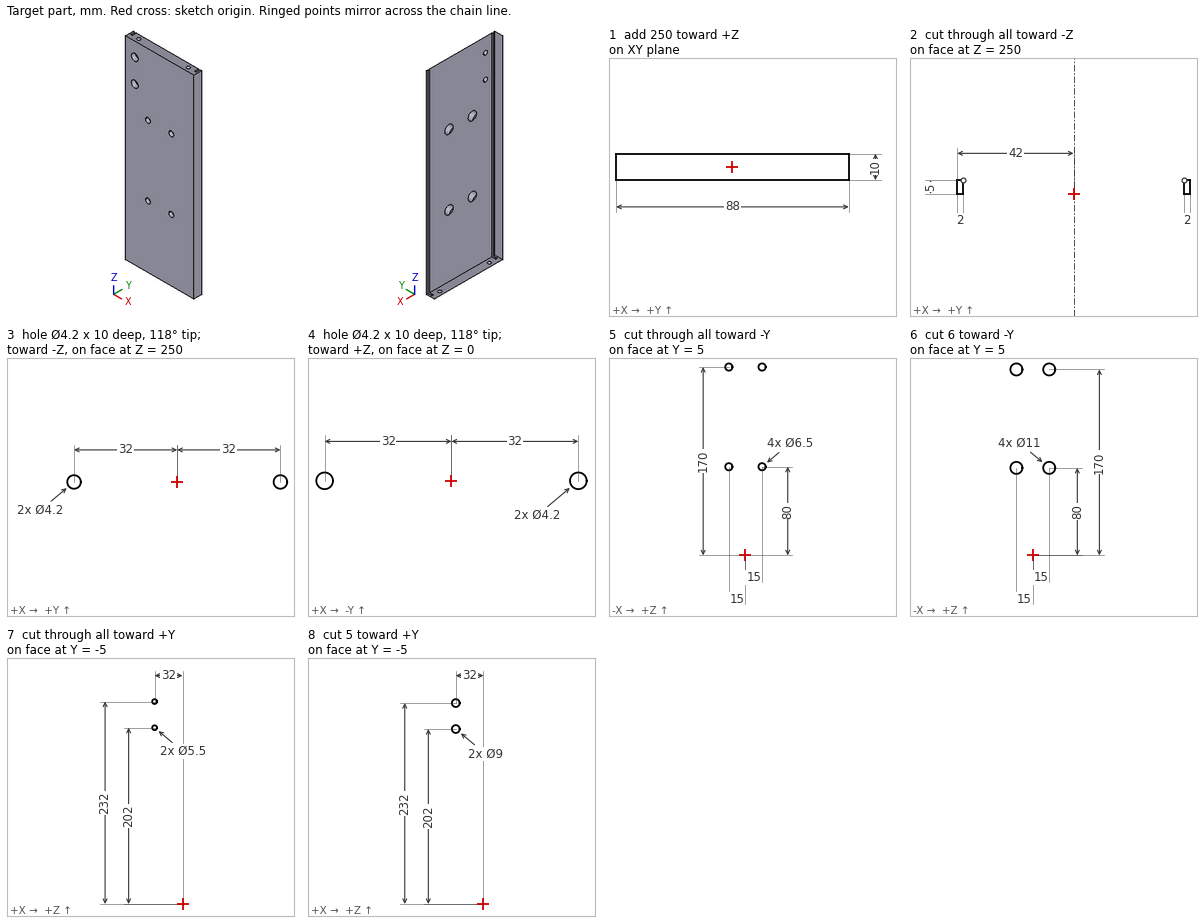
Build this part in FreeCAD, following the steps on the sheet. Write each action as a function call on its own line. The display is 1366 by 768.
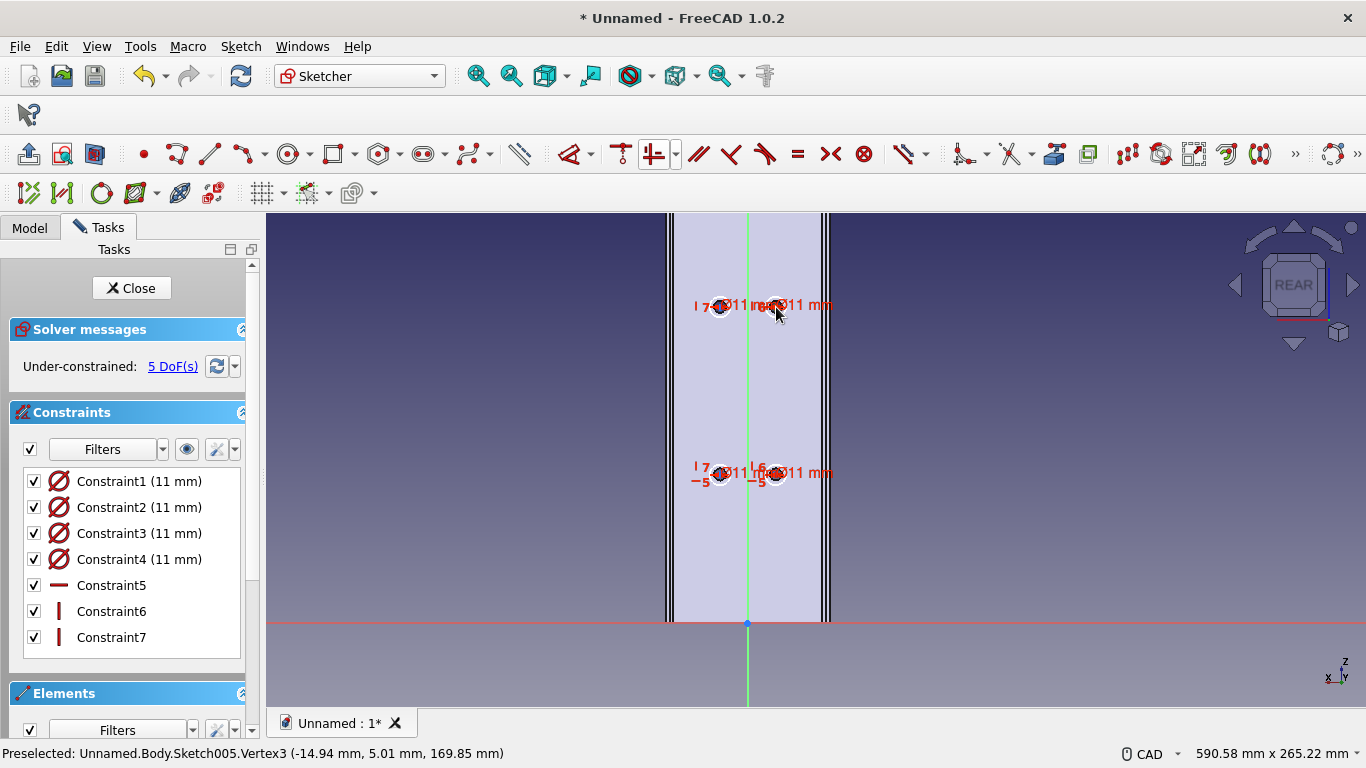
click(720, 307)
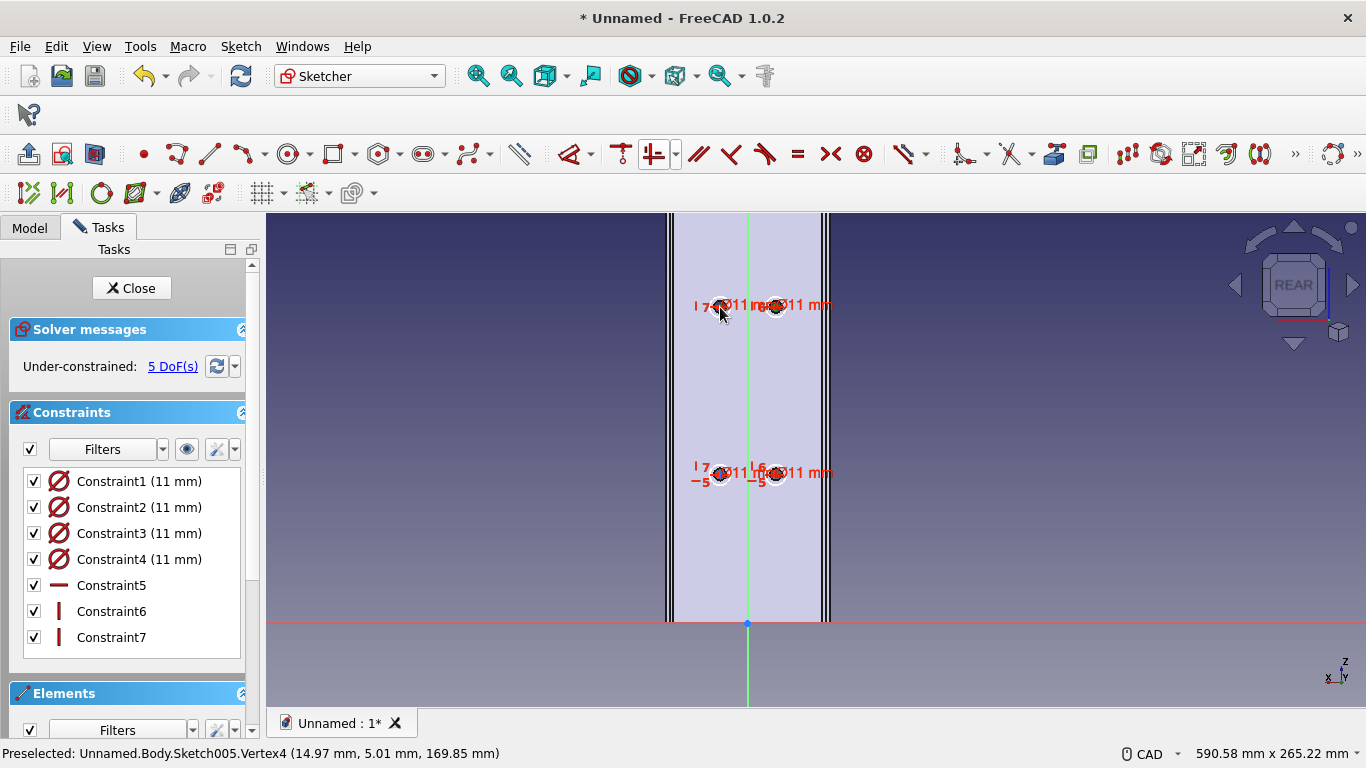
key(h)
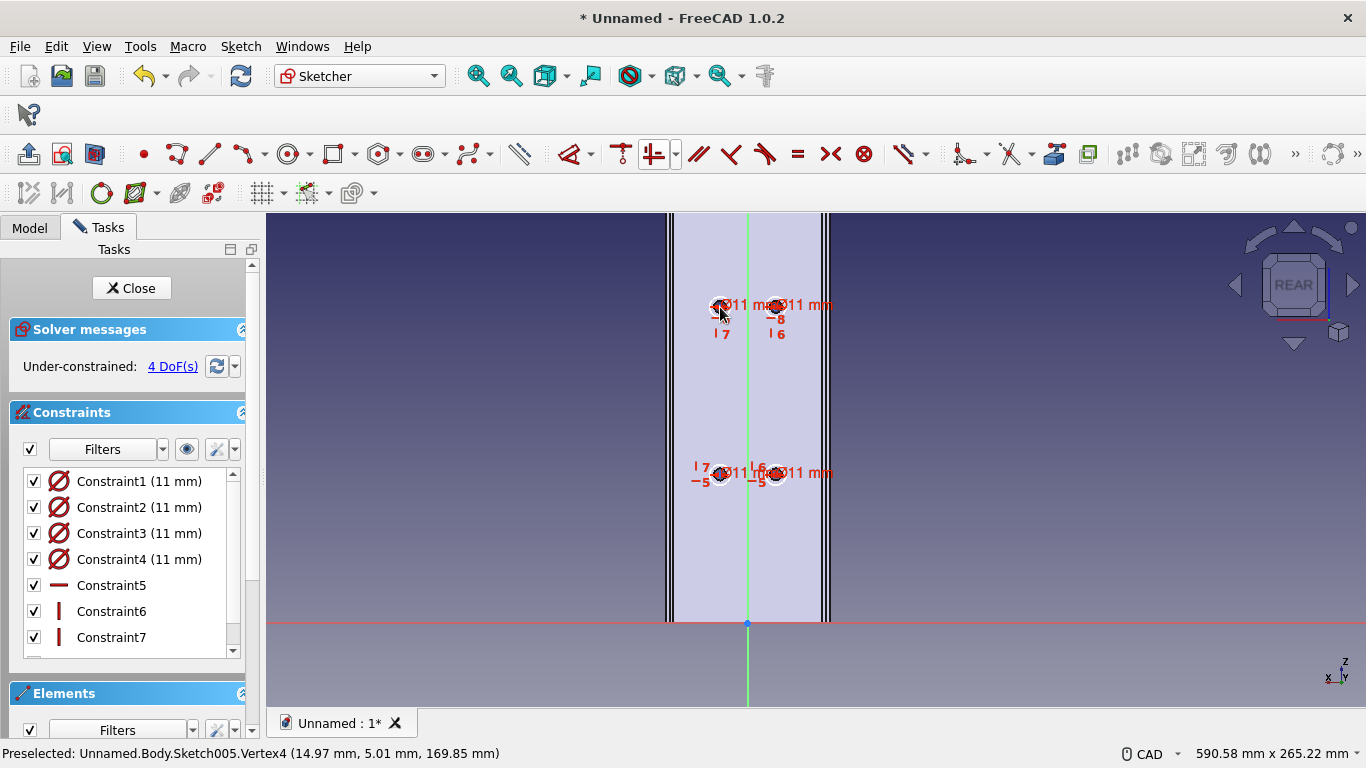
click(568, 154)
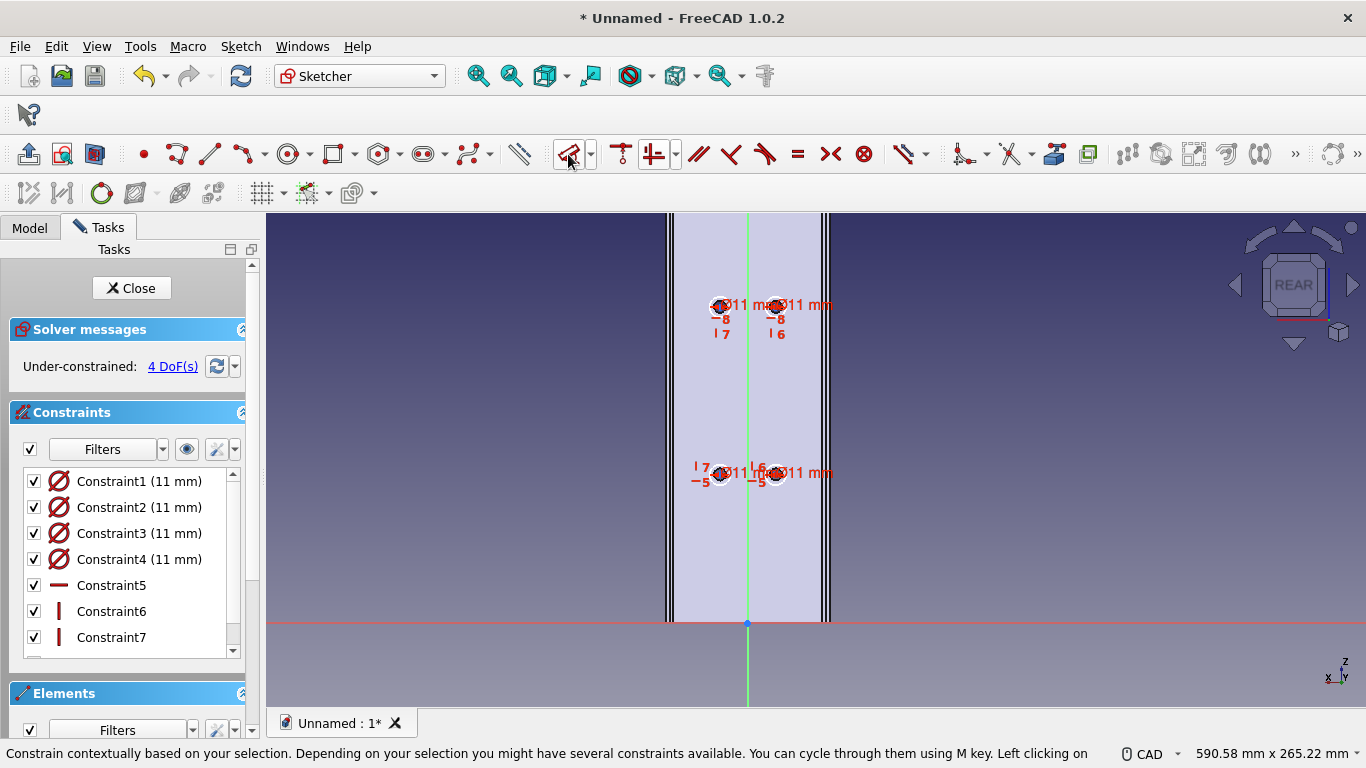
scroll(776, 475, up, 2)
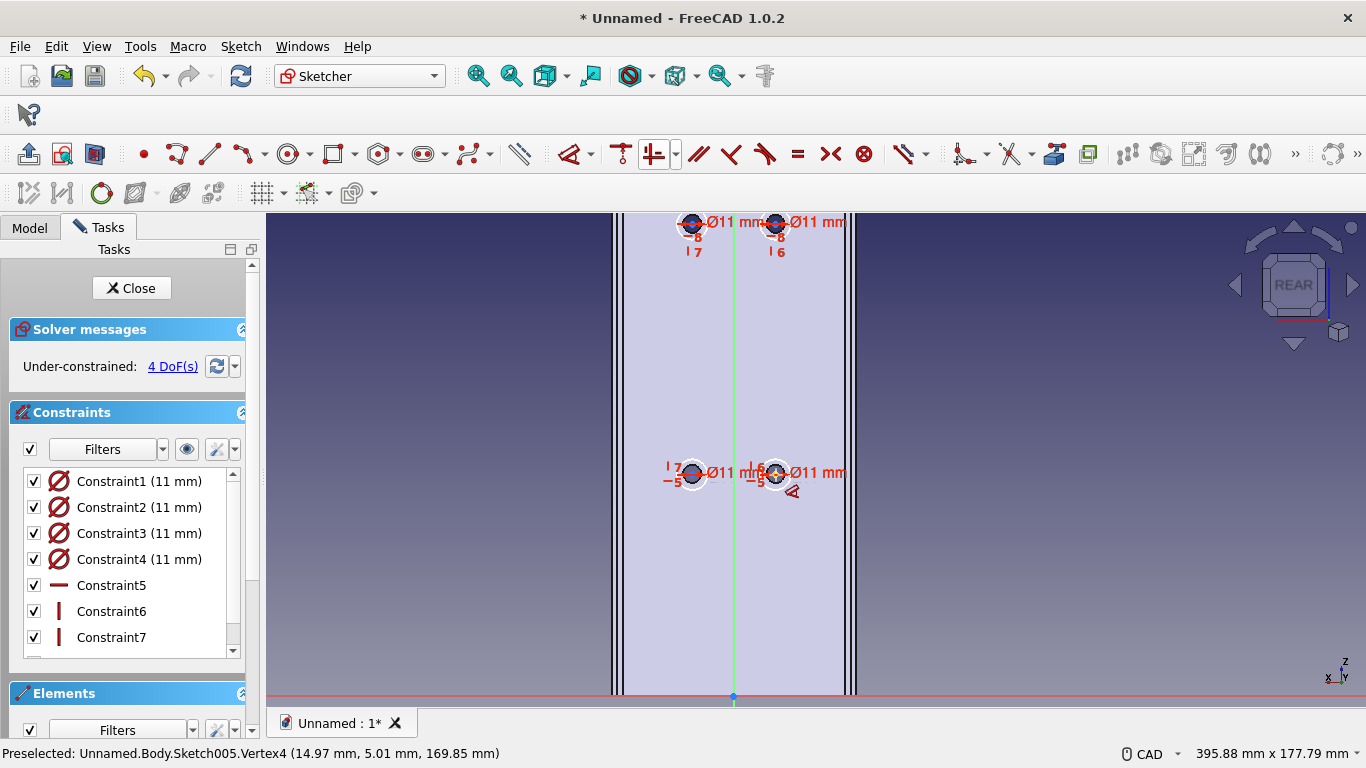
click(775, 475)
click(755, 441)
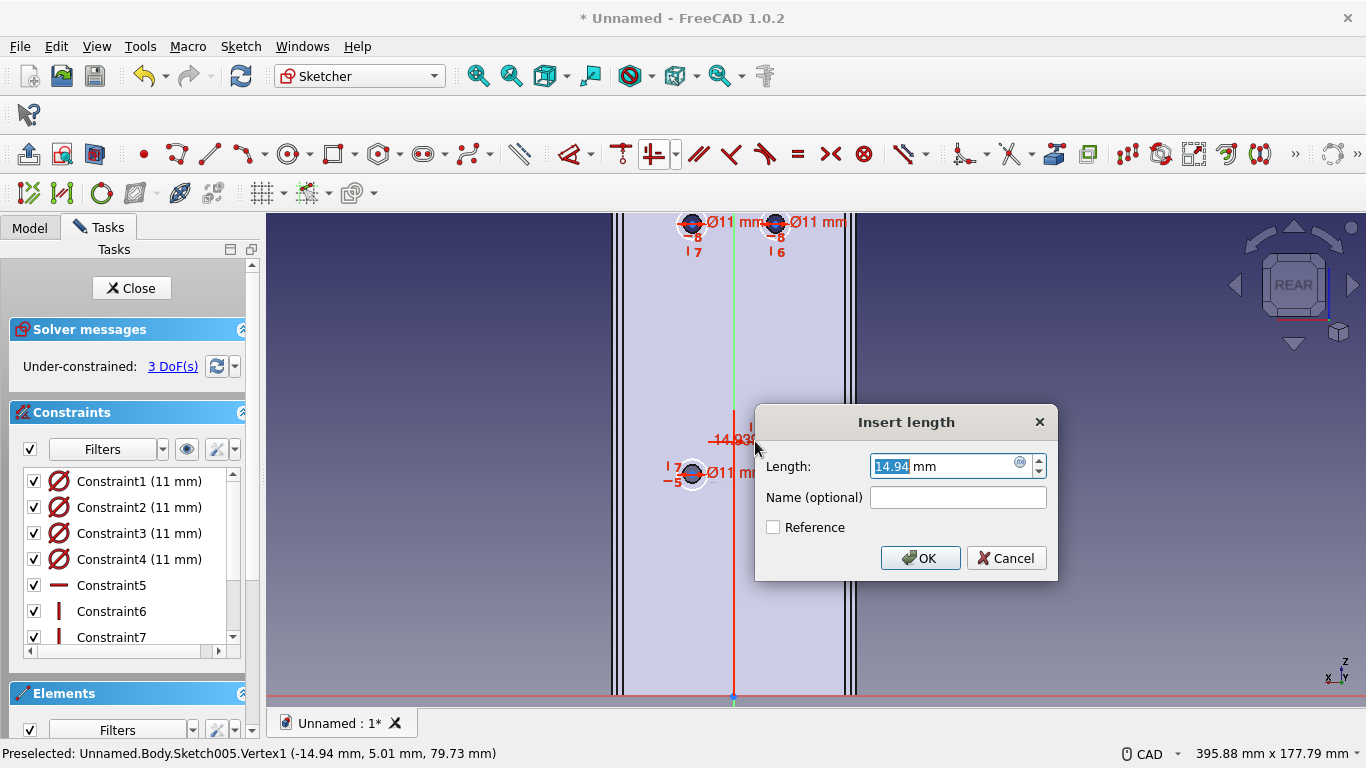
text(15)
key(Return)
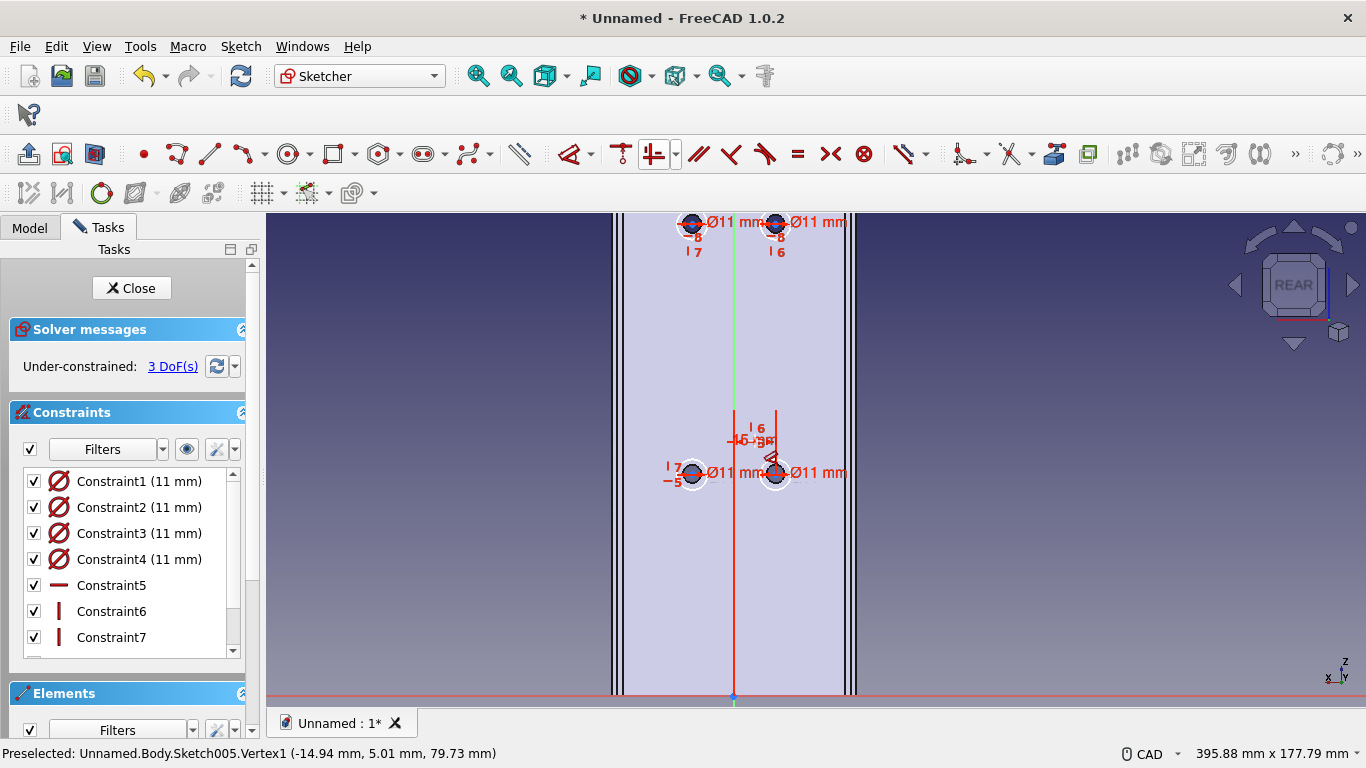
click(776, 475)
click(810, 577)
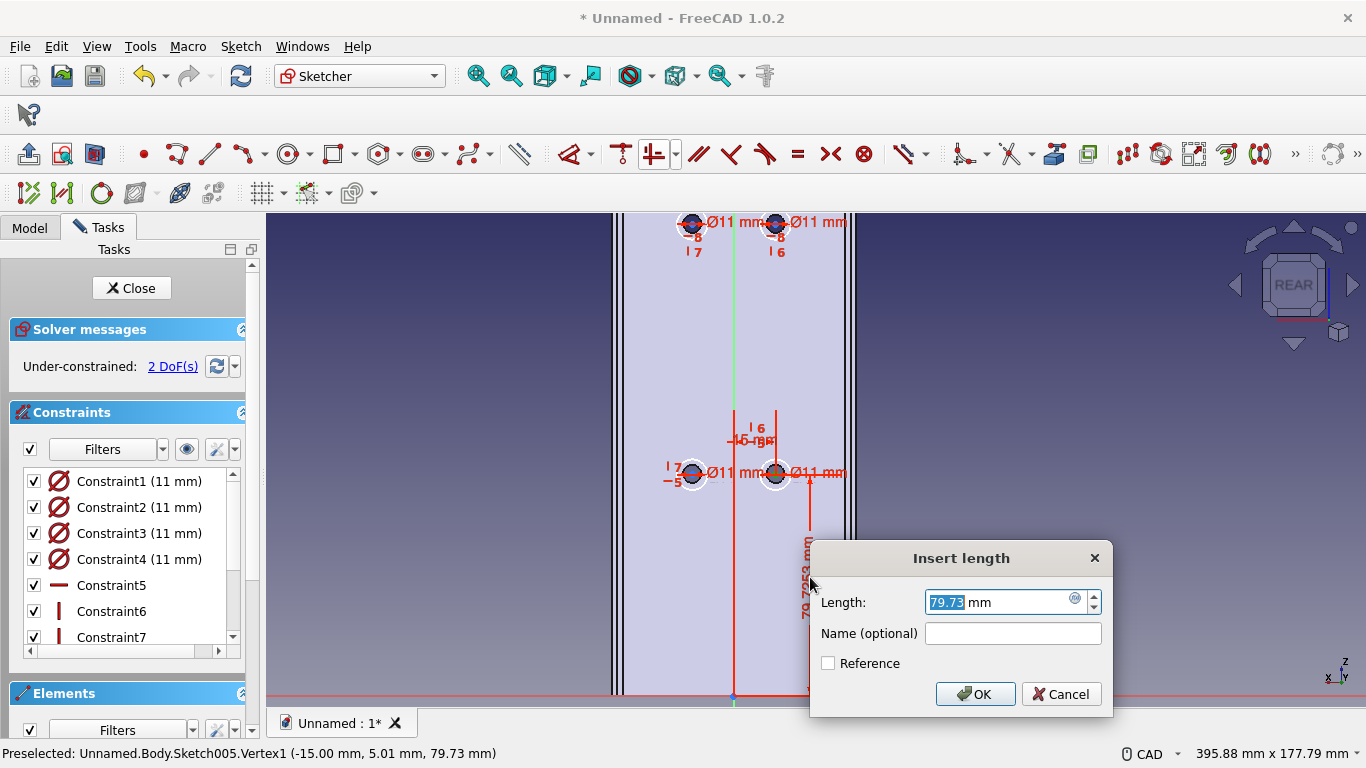
text(80)
key(Return)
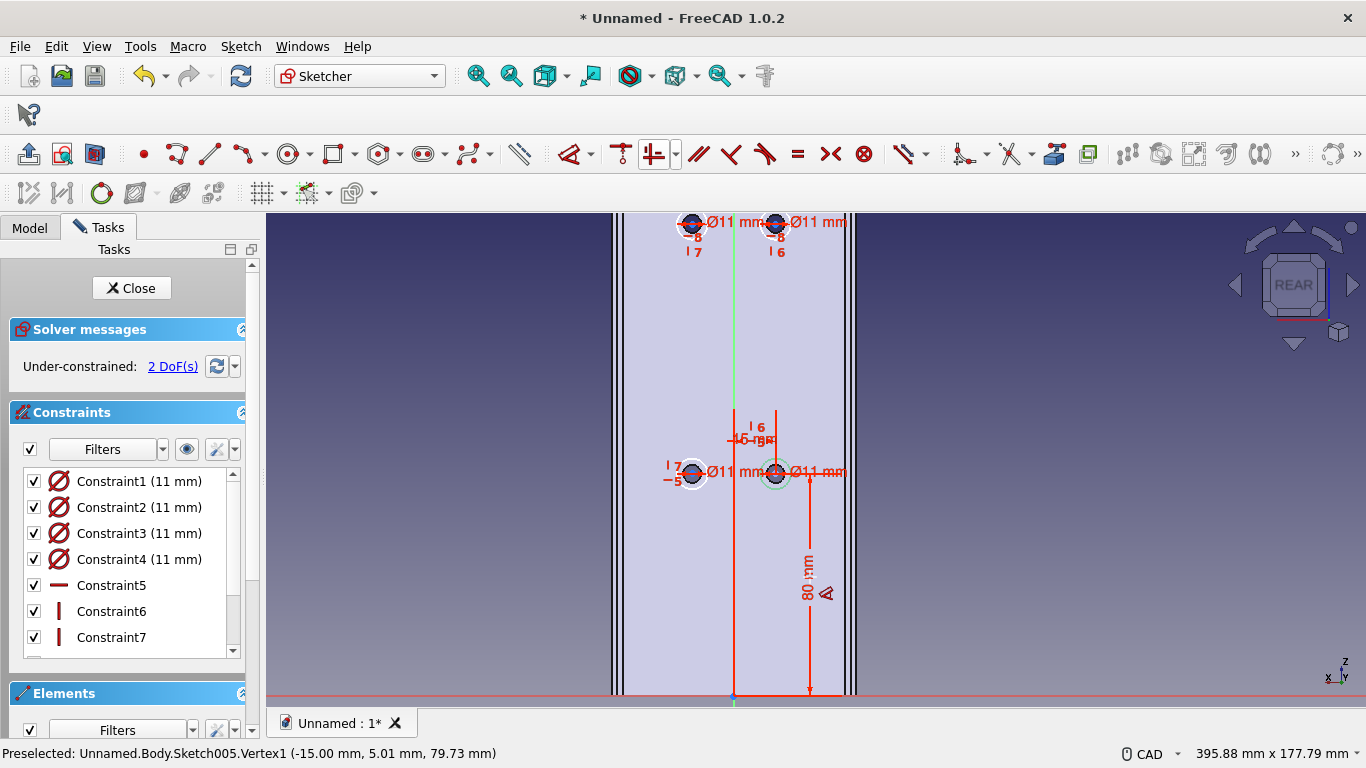
click(692, 474)
click(713, 416)